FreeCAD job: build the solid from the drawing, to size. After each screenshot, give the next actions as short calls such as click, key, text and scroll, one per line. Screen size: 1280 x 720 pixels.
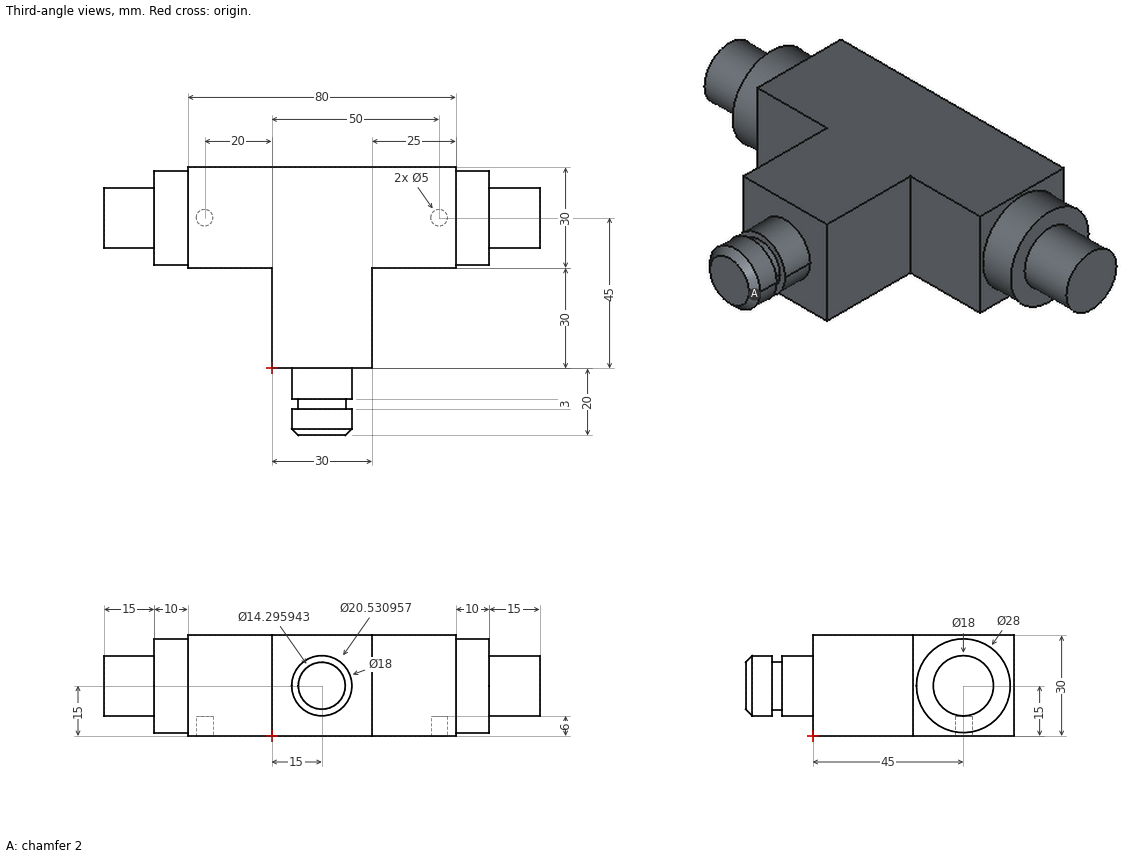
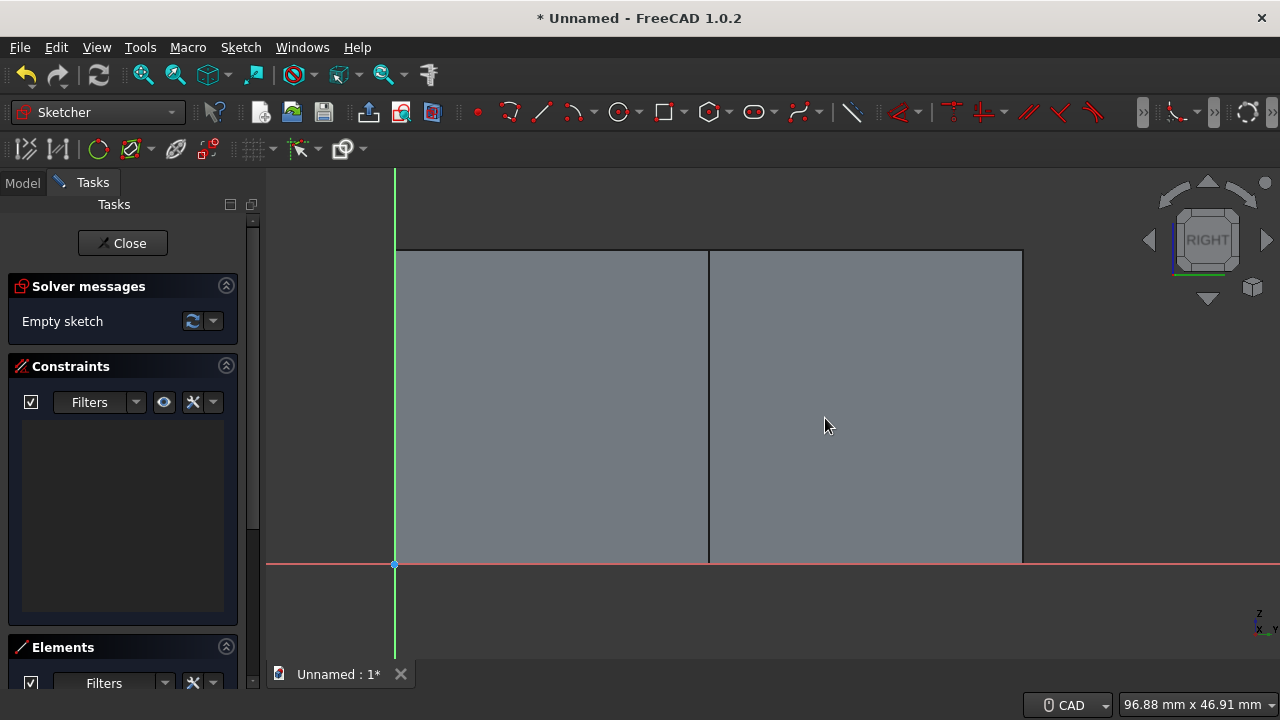
key(g)
key(c)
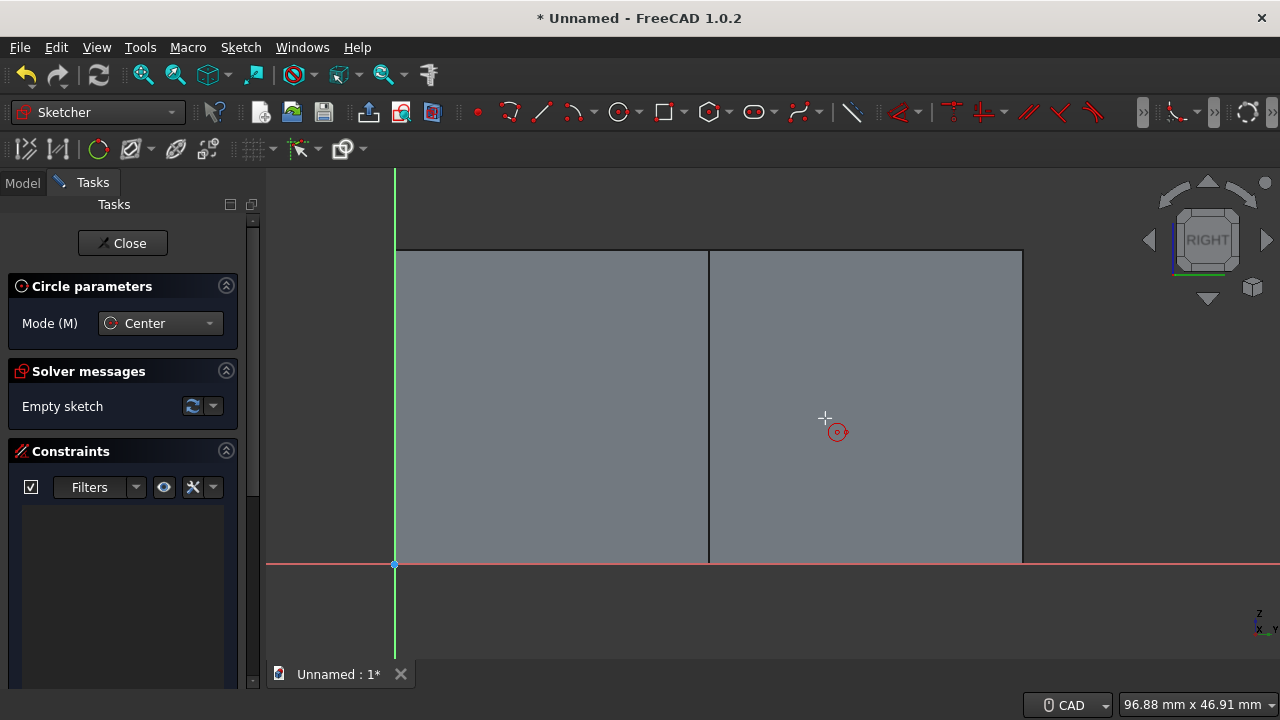
click(866, 407)
move(969, 304)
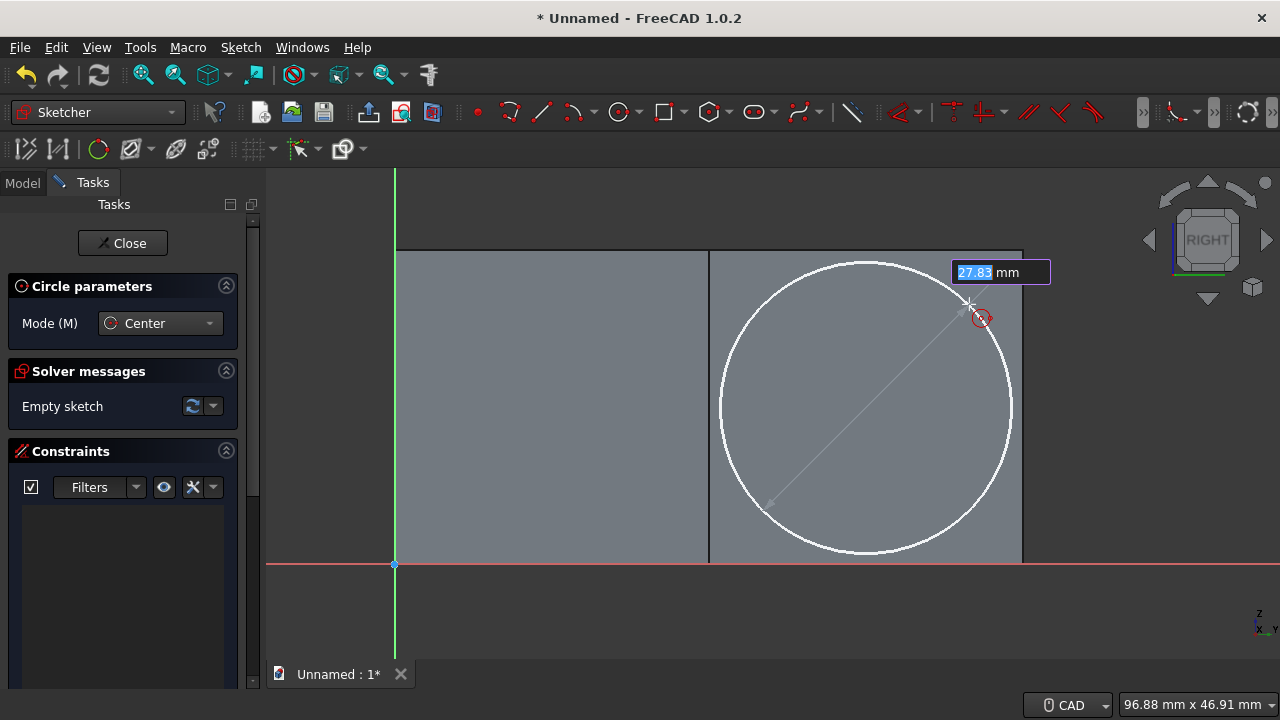
text(28)
key(Return)
key(Escape)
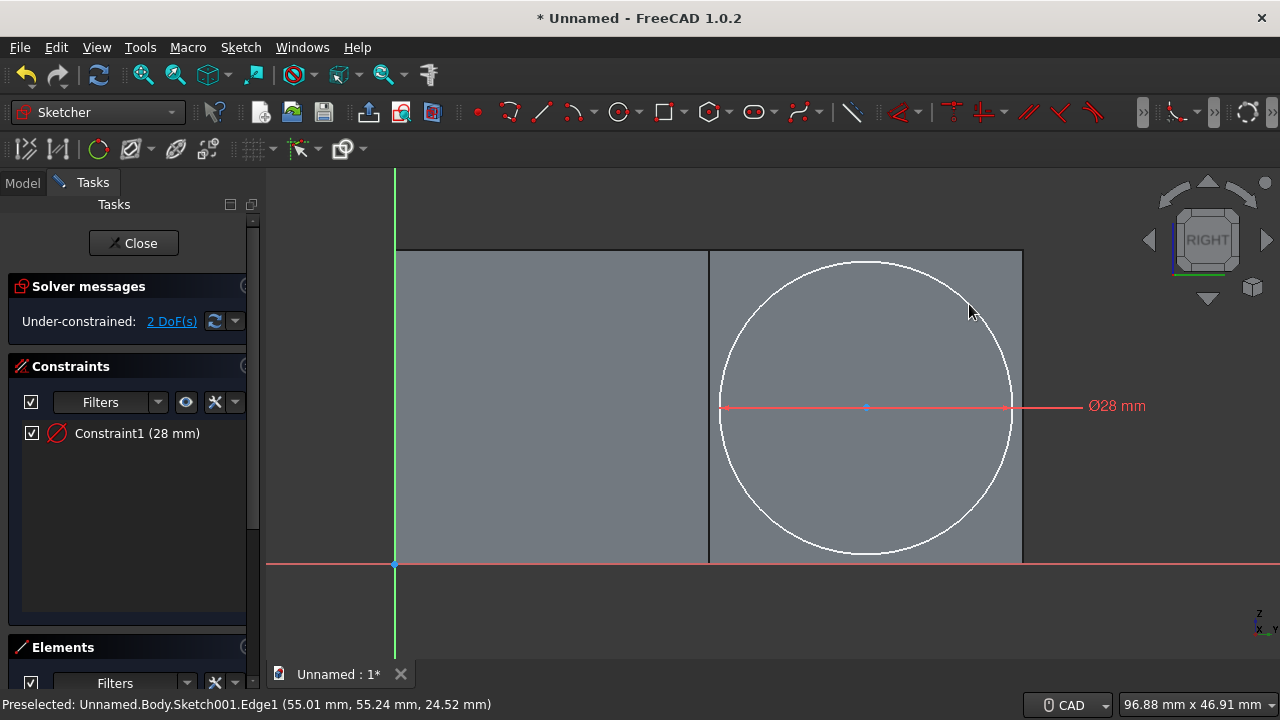
key(d)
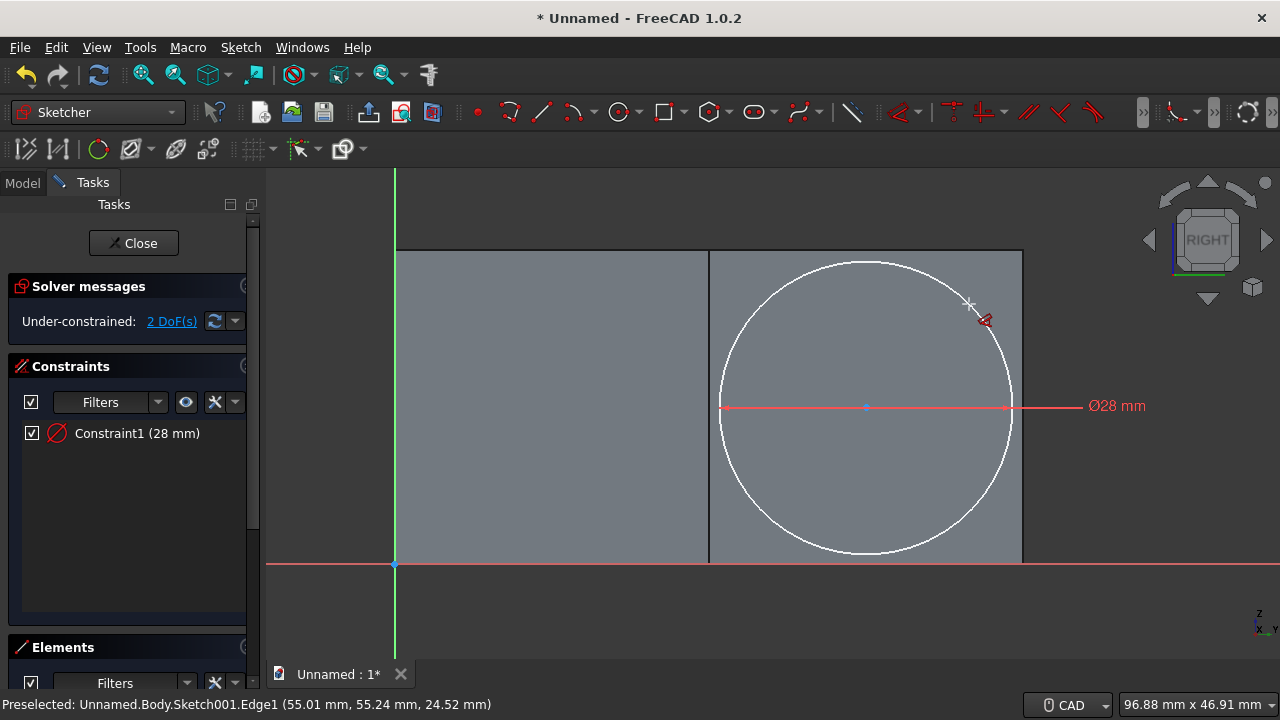
click(866, 408)
click(630, 598)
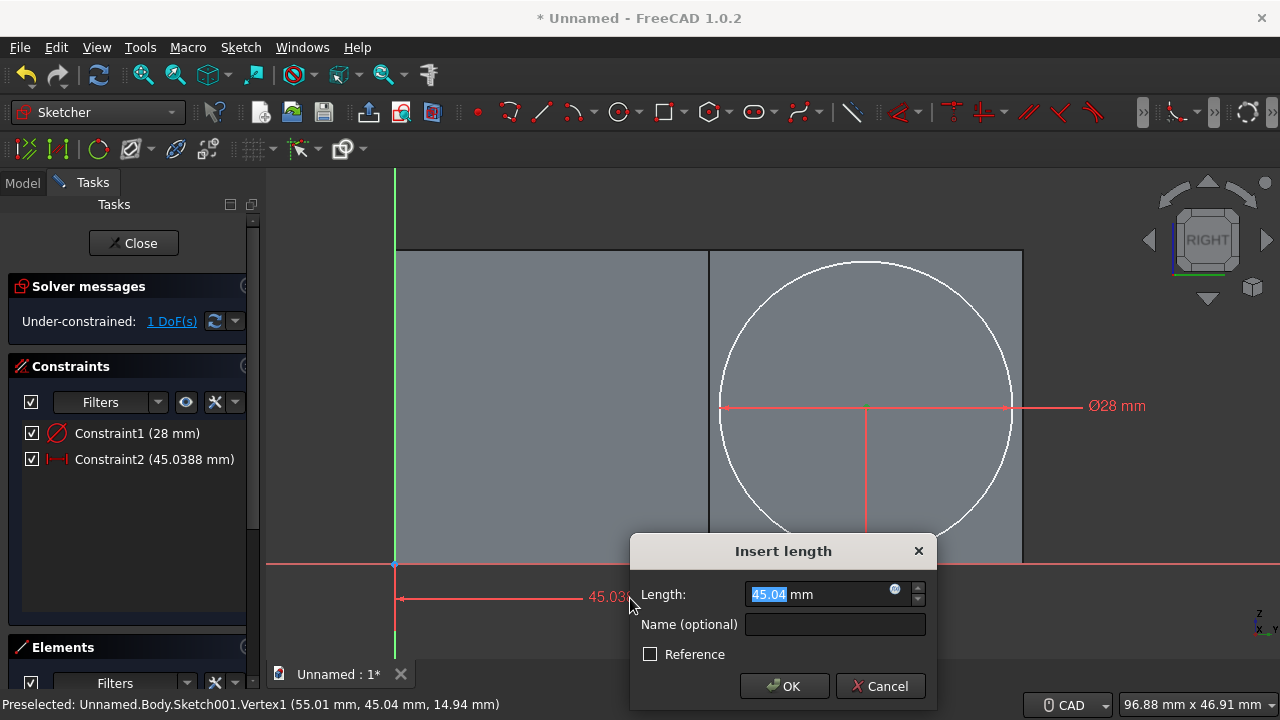
text(45)
key(Return)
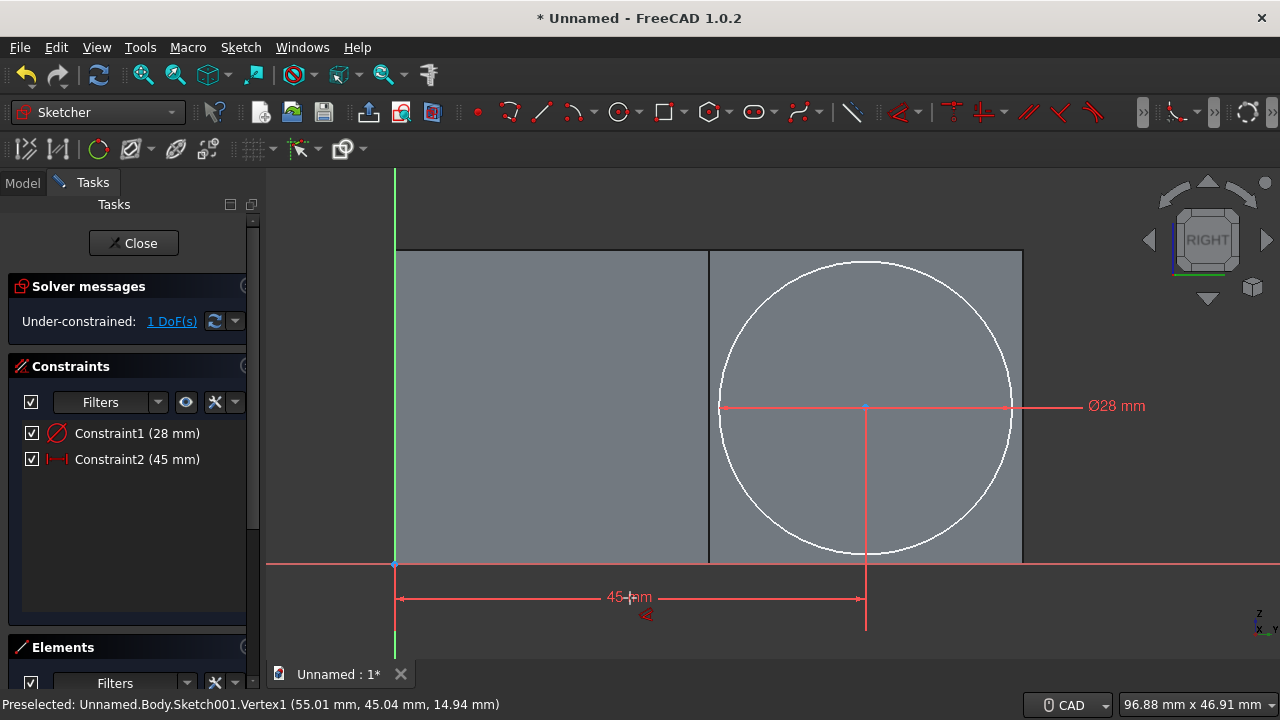
click(866, 408)
click(361, 486)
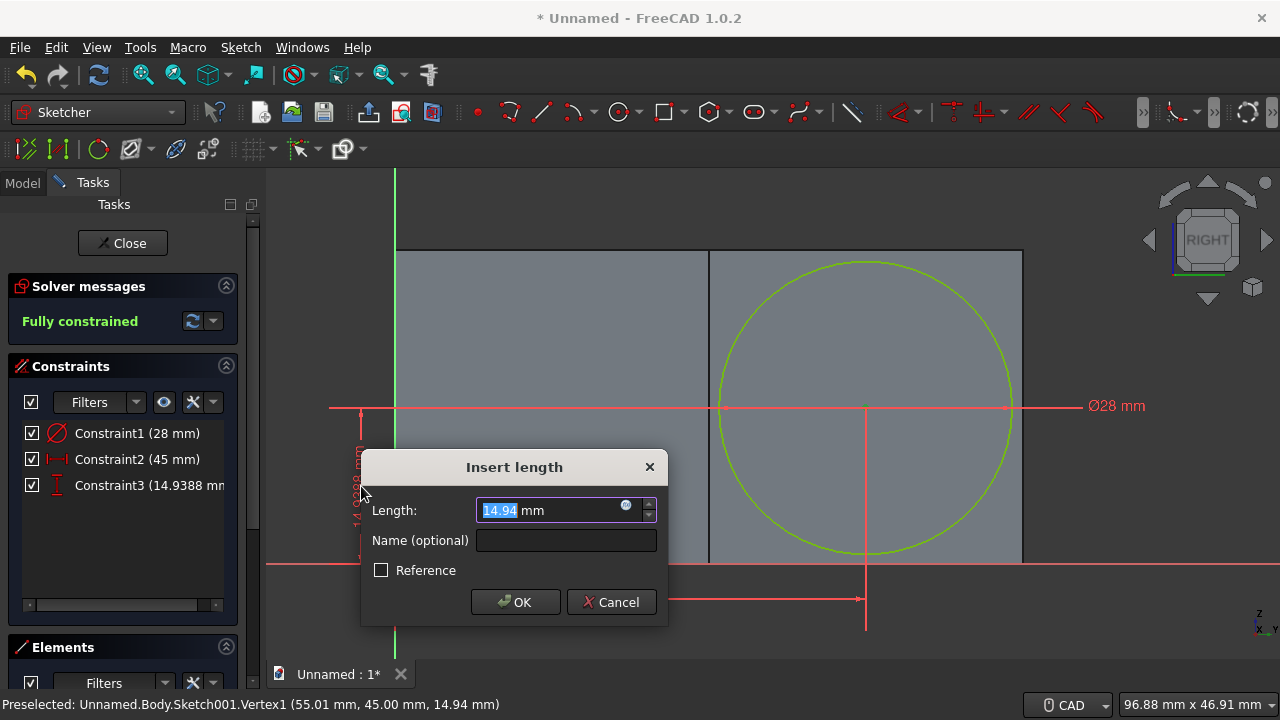
text(15)
key(Return)
key(Escape)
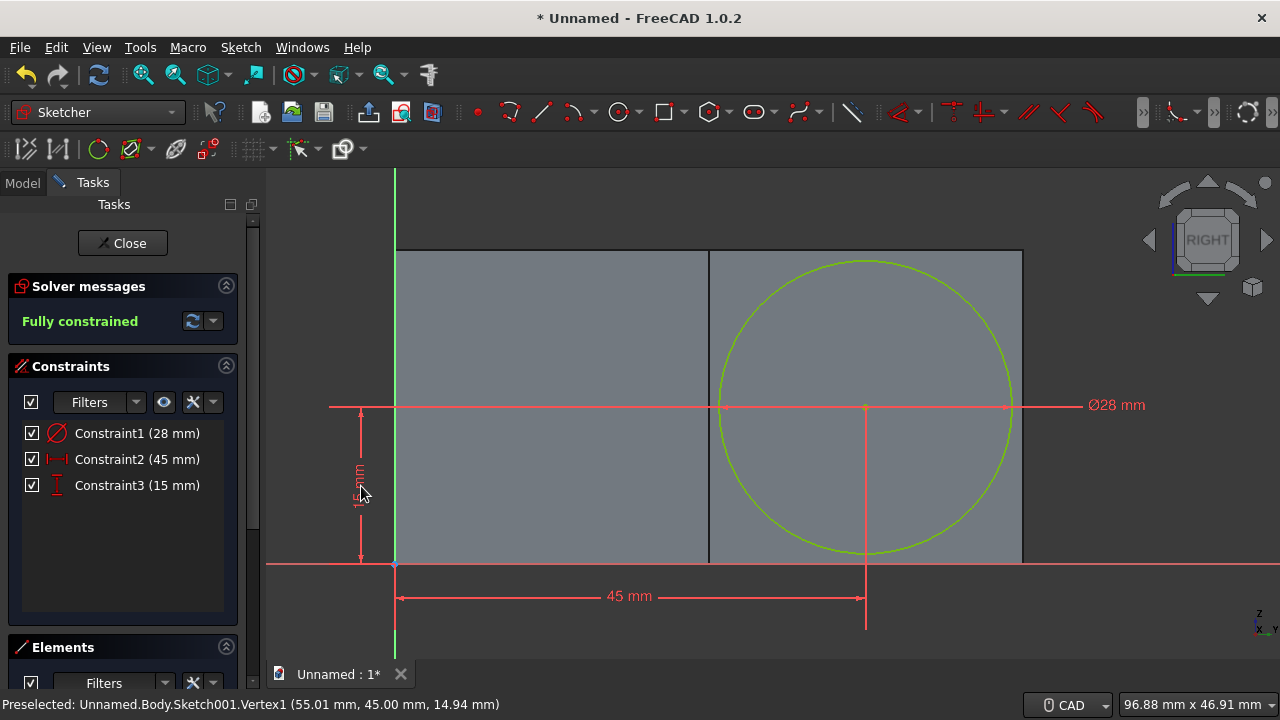
click(123, 243)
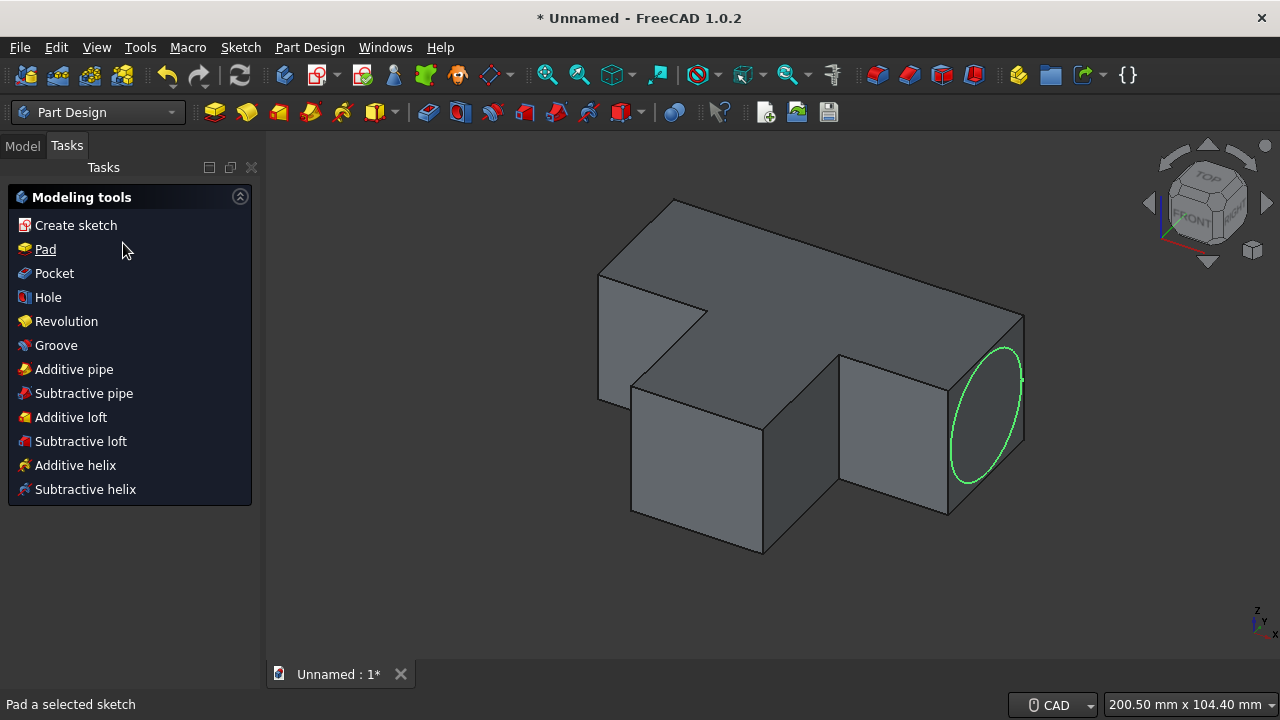
click(216, 112)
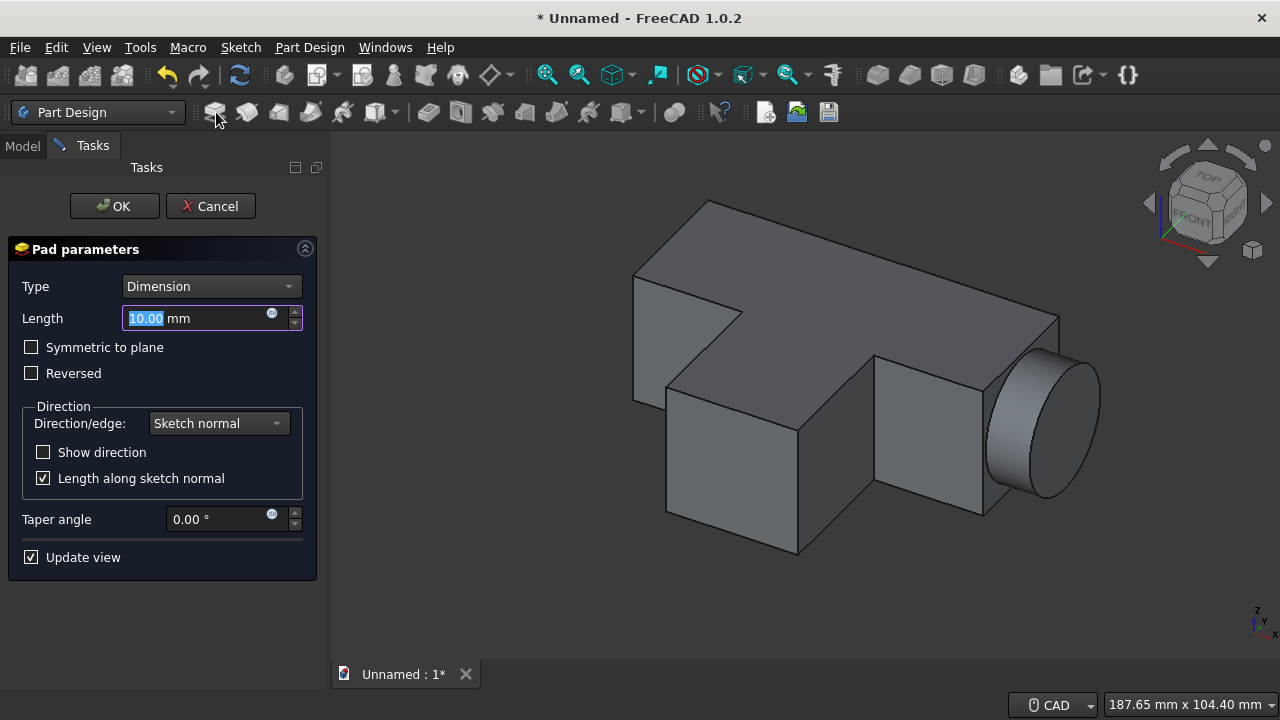
text(10)
key(Tab)